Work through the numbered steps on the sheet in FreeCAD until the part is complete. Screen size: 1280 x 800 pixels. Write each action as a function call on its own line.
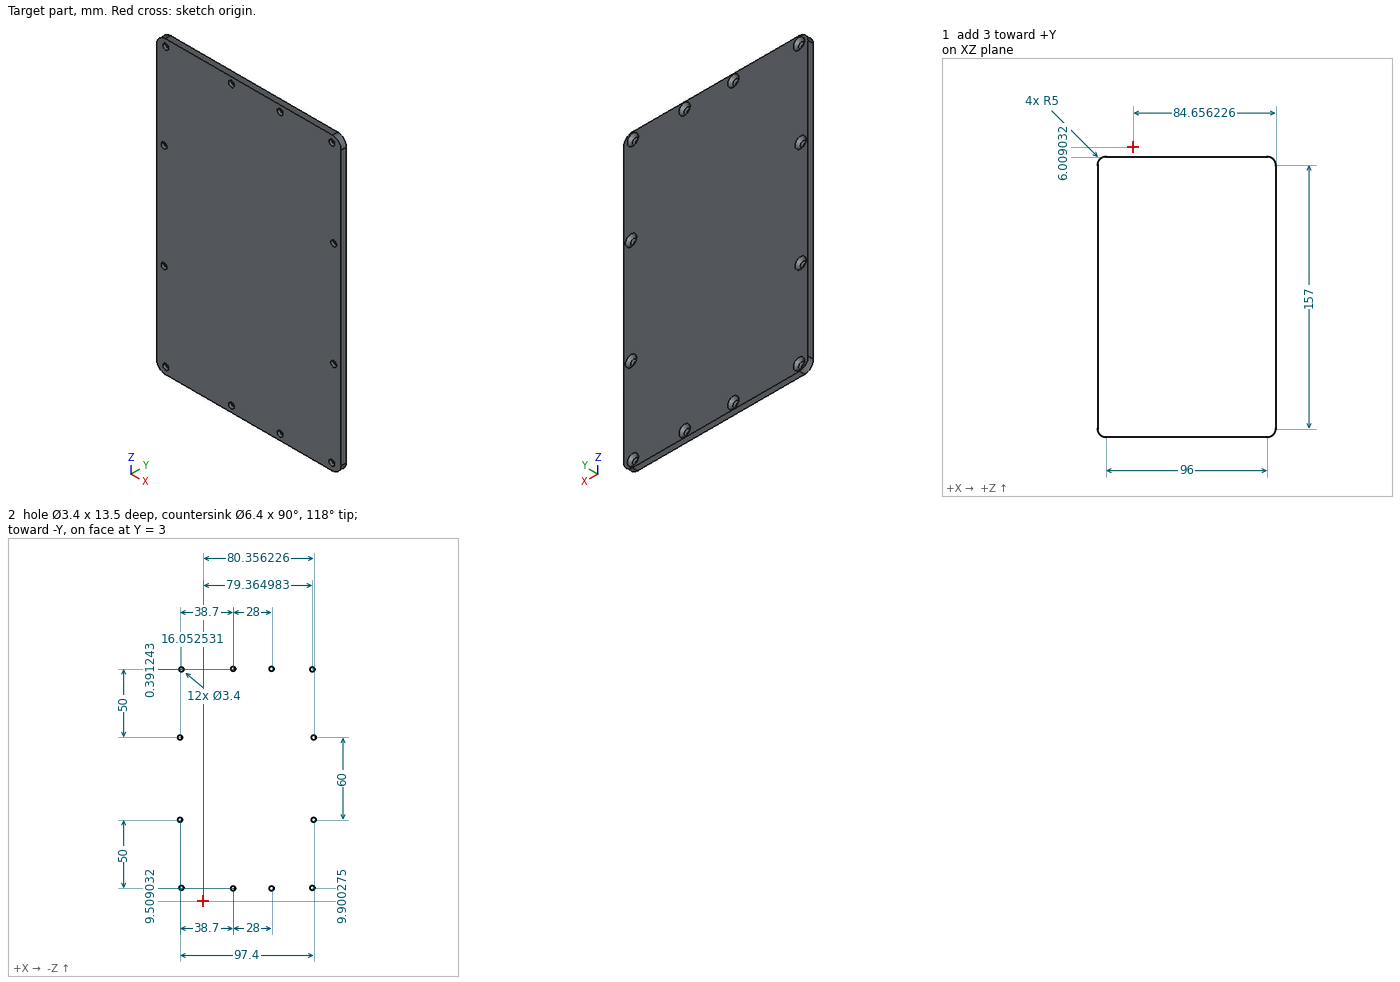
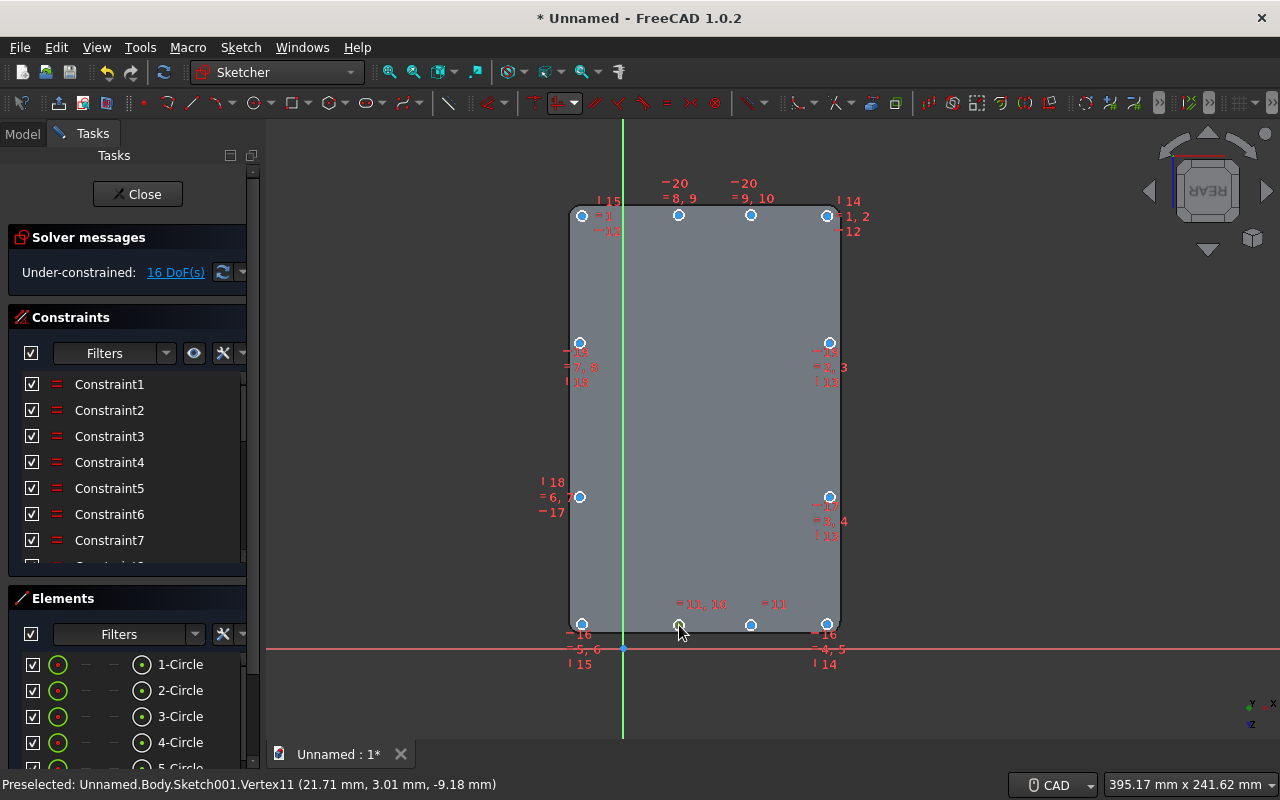
click(751, 625)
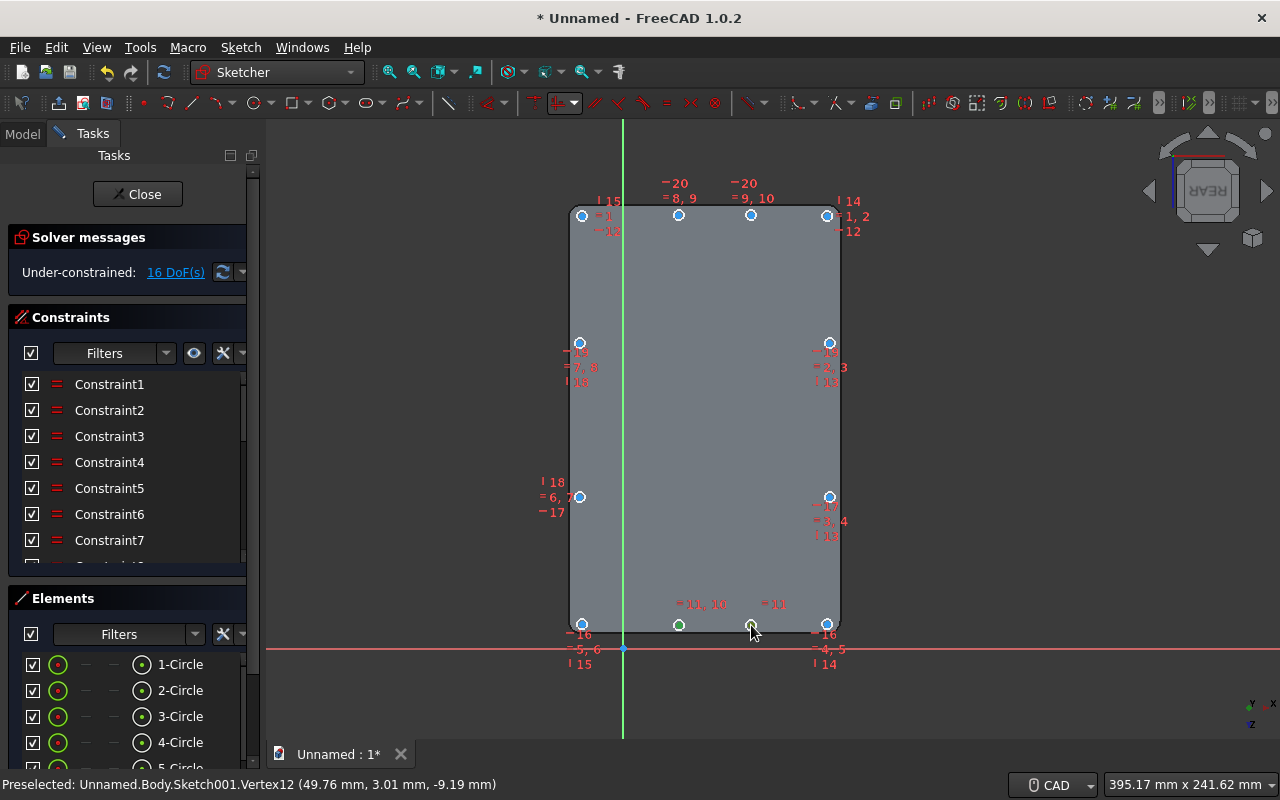
key(h)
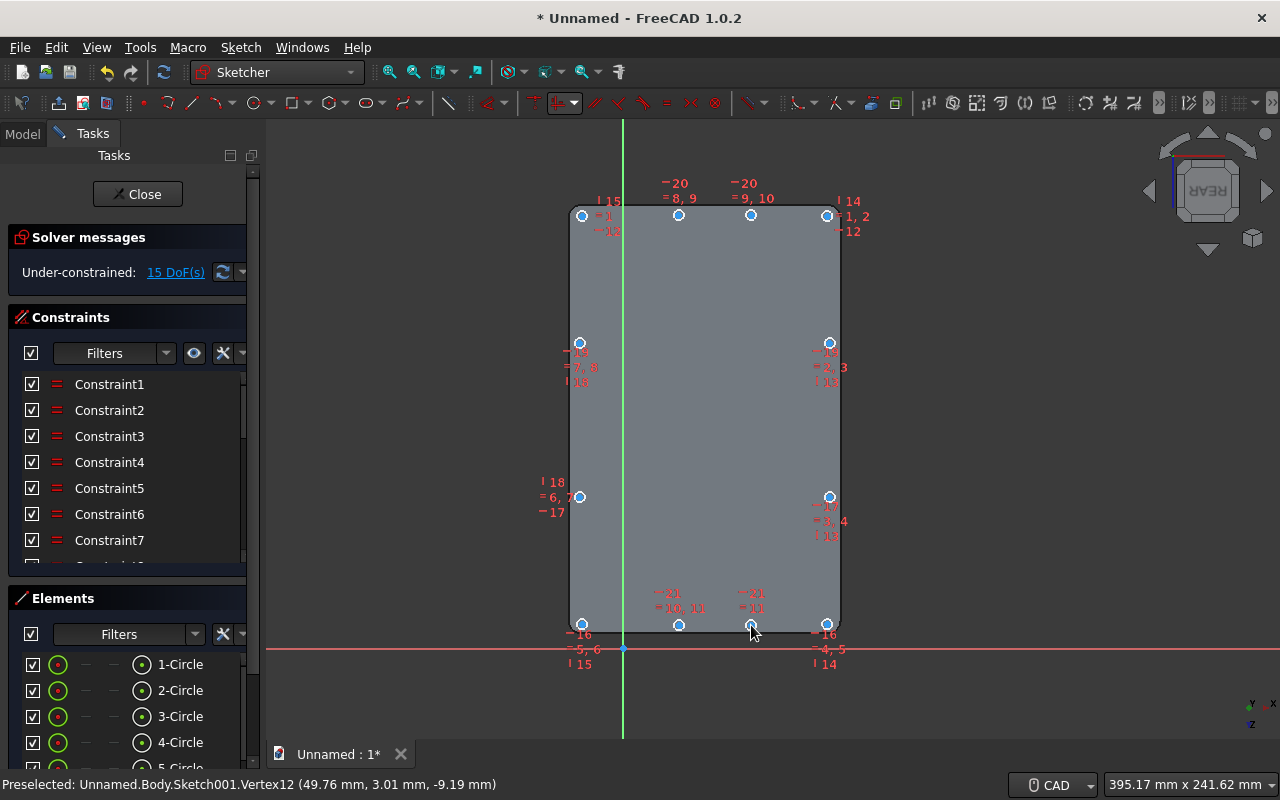
click(488, 104)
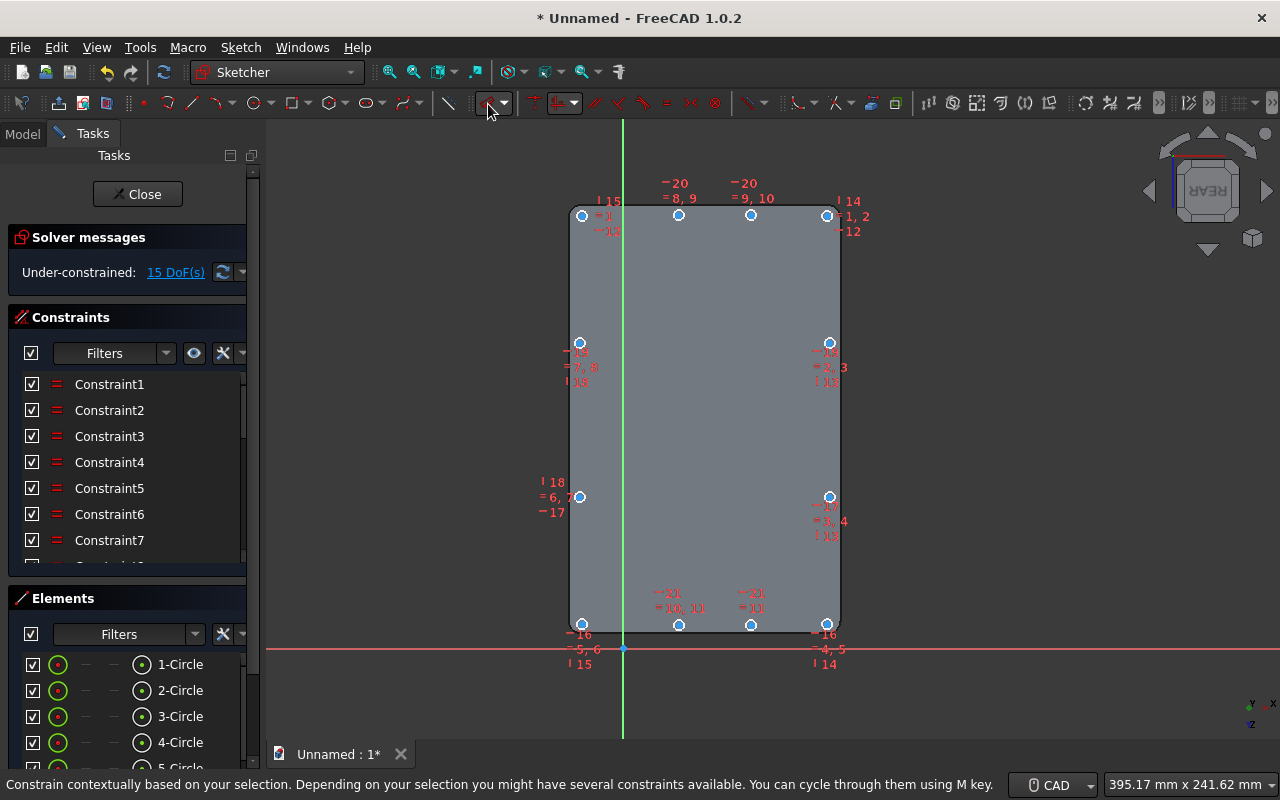
scroll(577, 216, up, 8)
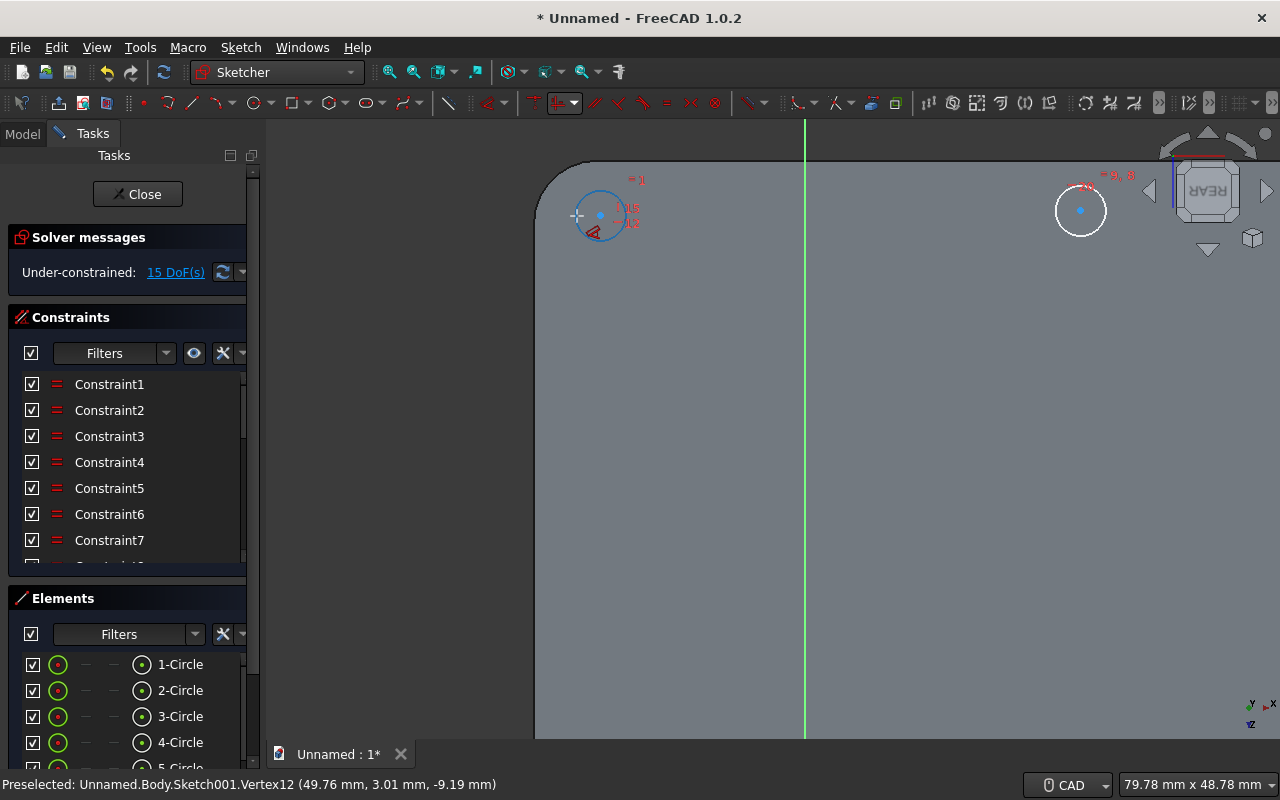
click(576, 215)
click(544, 214)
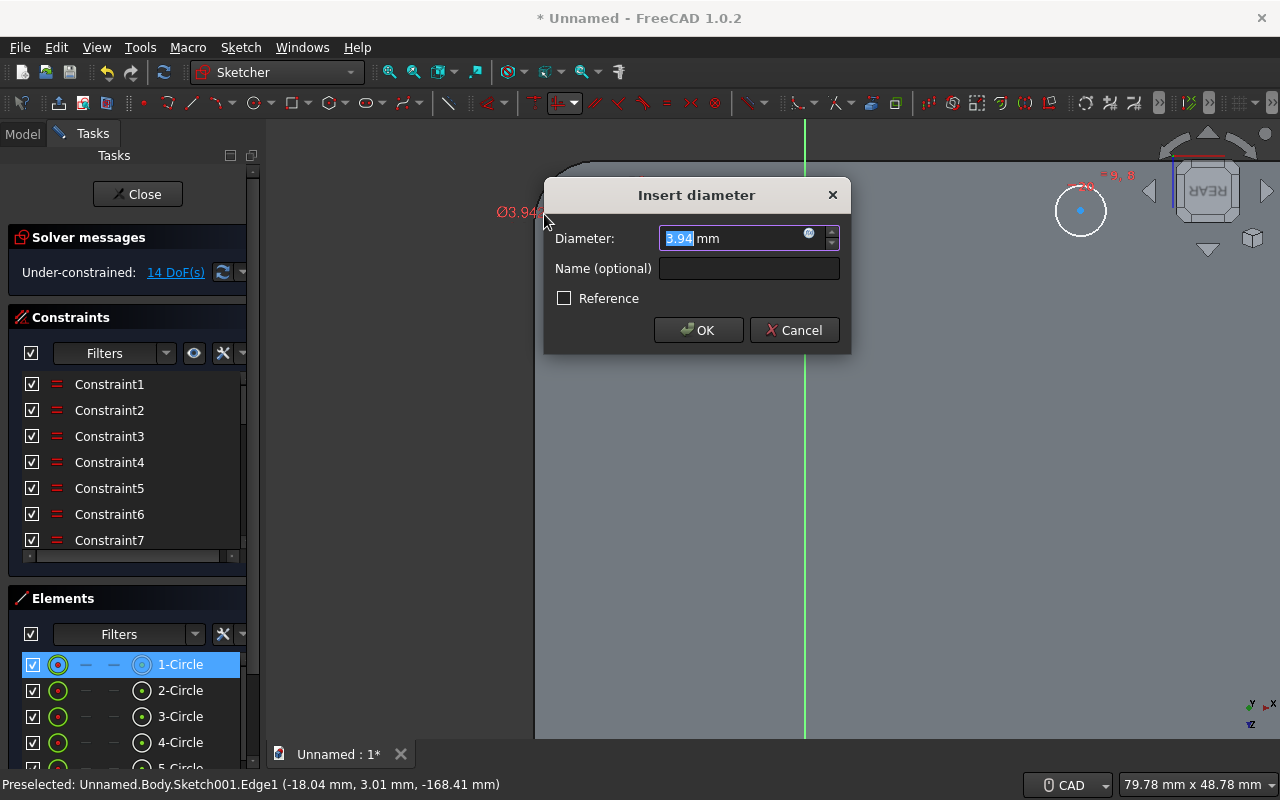
text(3.4)
key(Return)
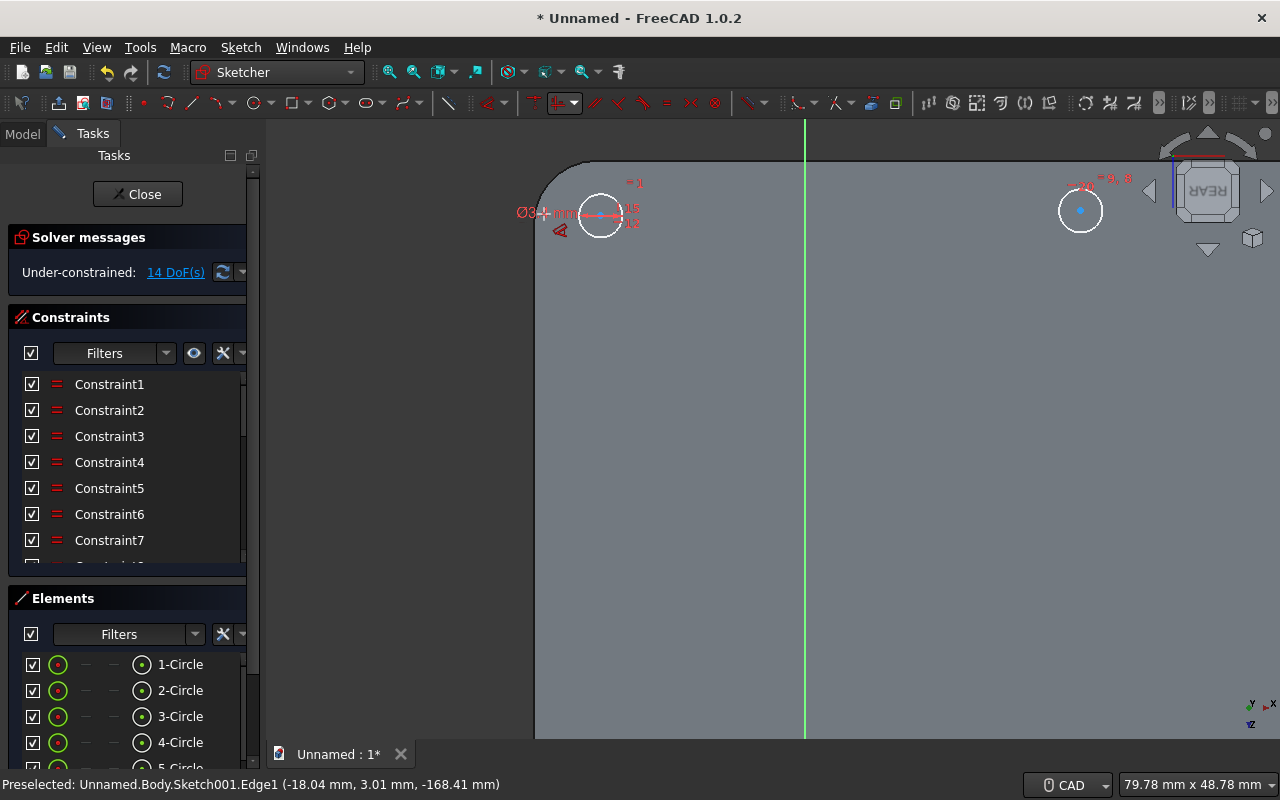
scroll(577, 216, down, 8)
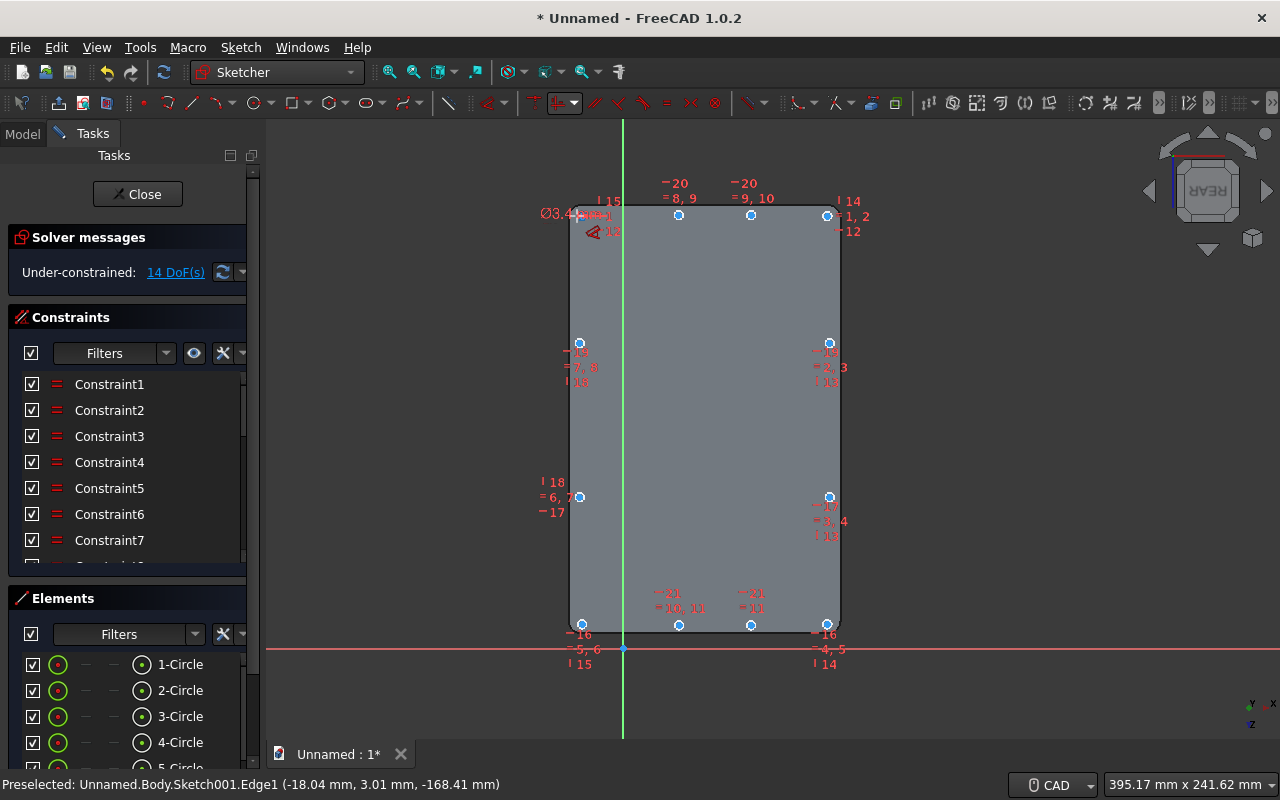
click(830, 343)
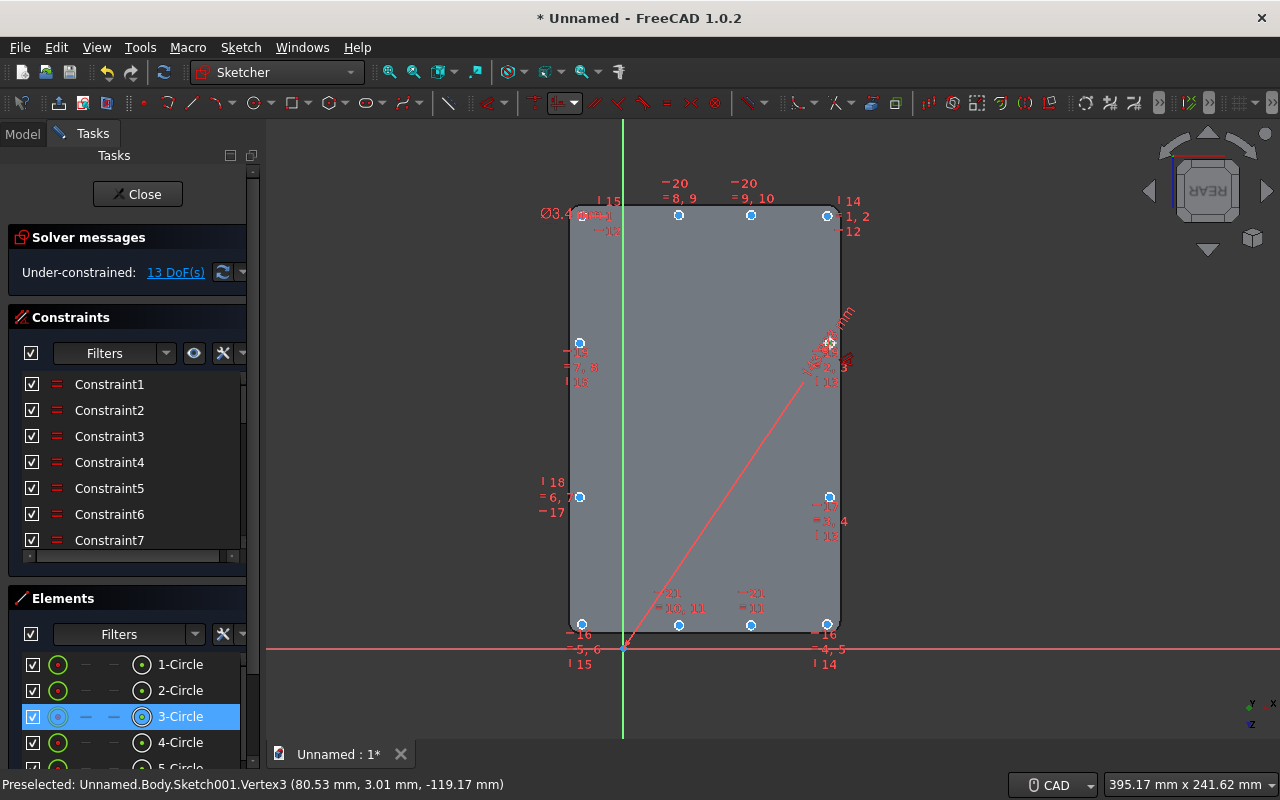
click(830, 497)
click(864, 420)